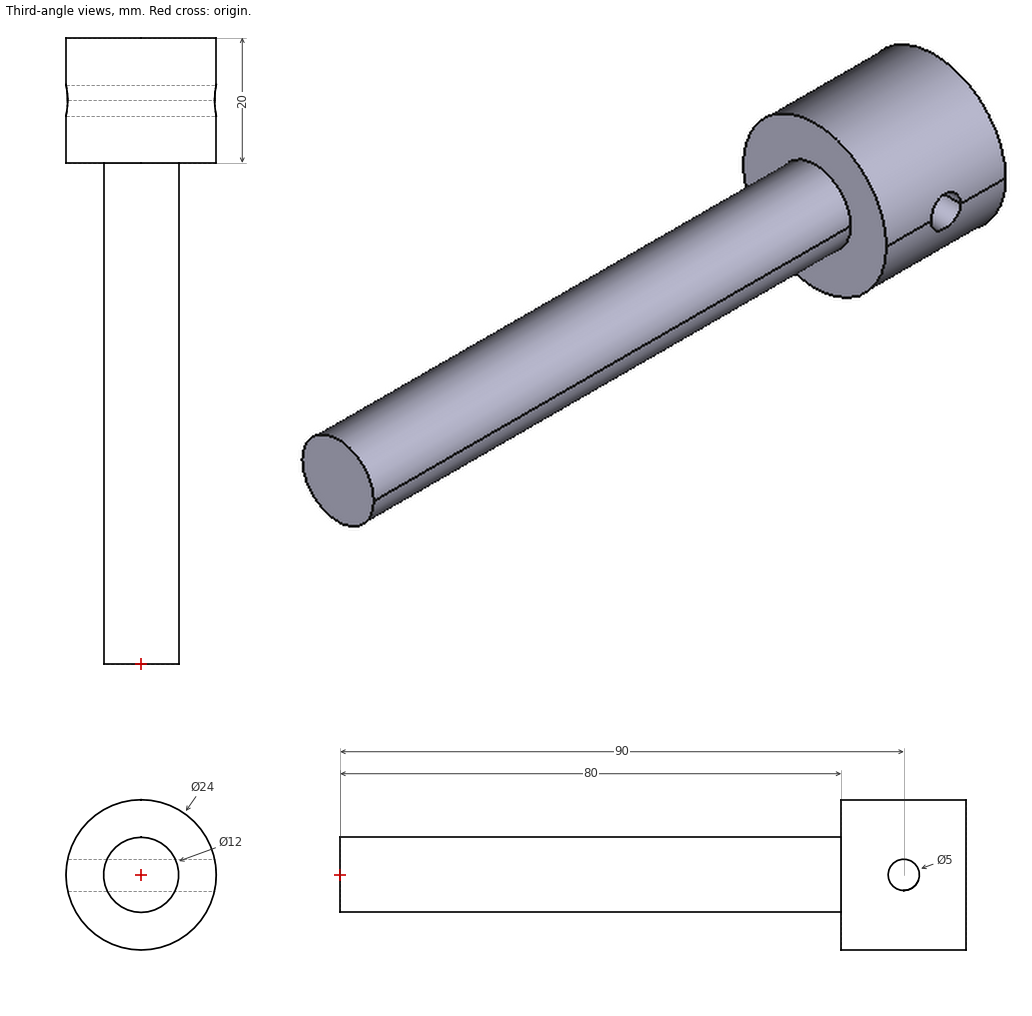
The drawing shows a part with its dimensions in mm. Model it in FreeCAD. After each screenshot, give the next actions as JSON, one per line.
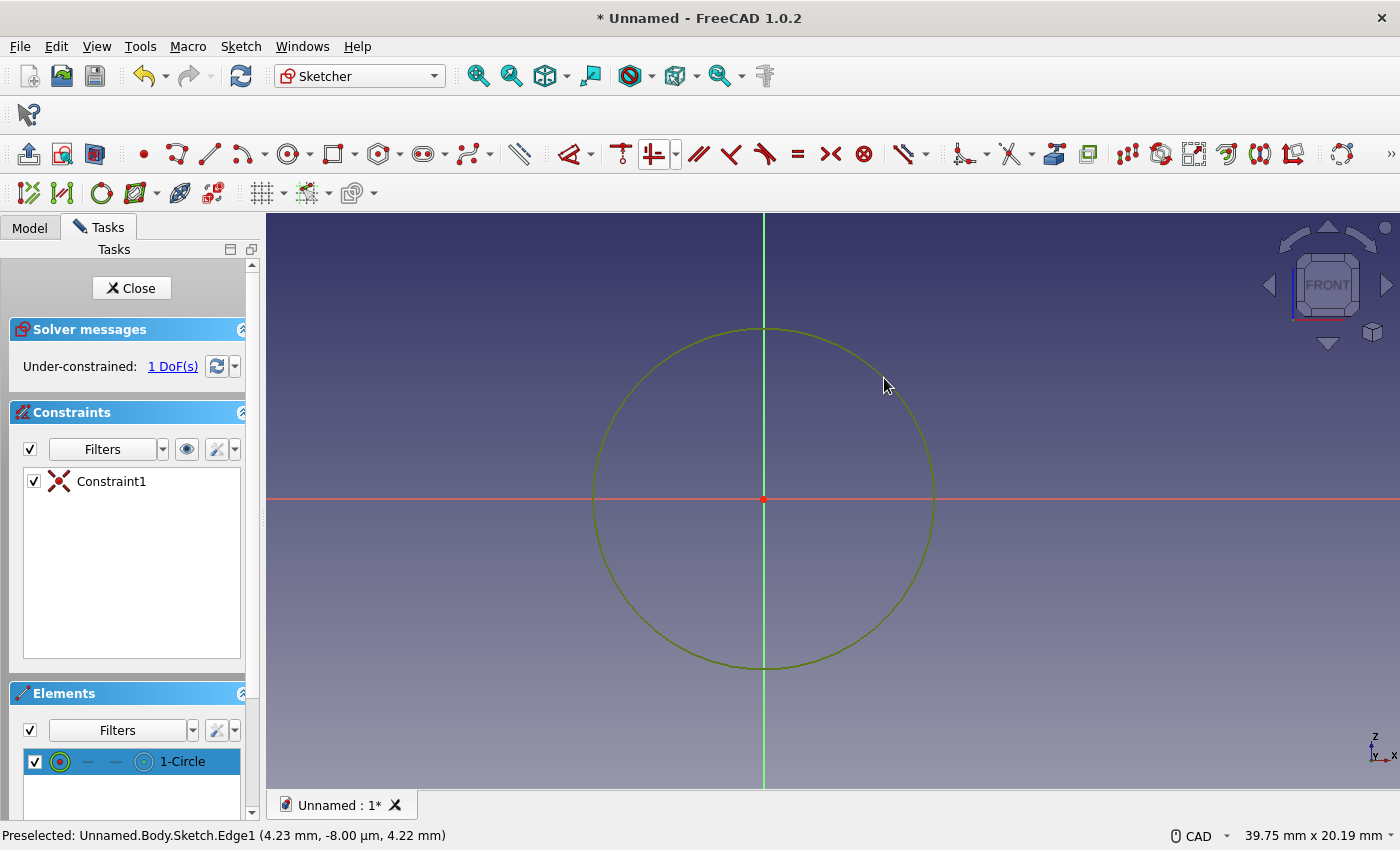
{"action": "key", "text": "k o"}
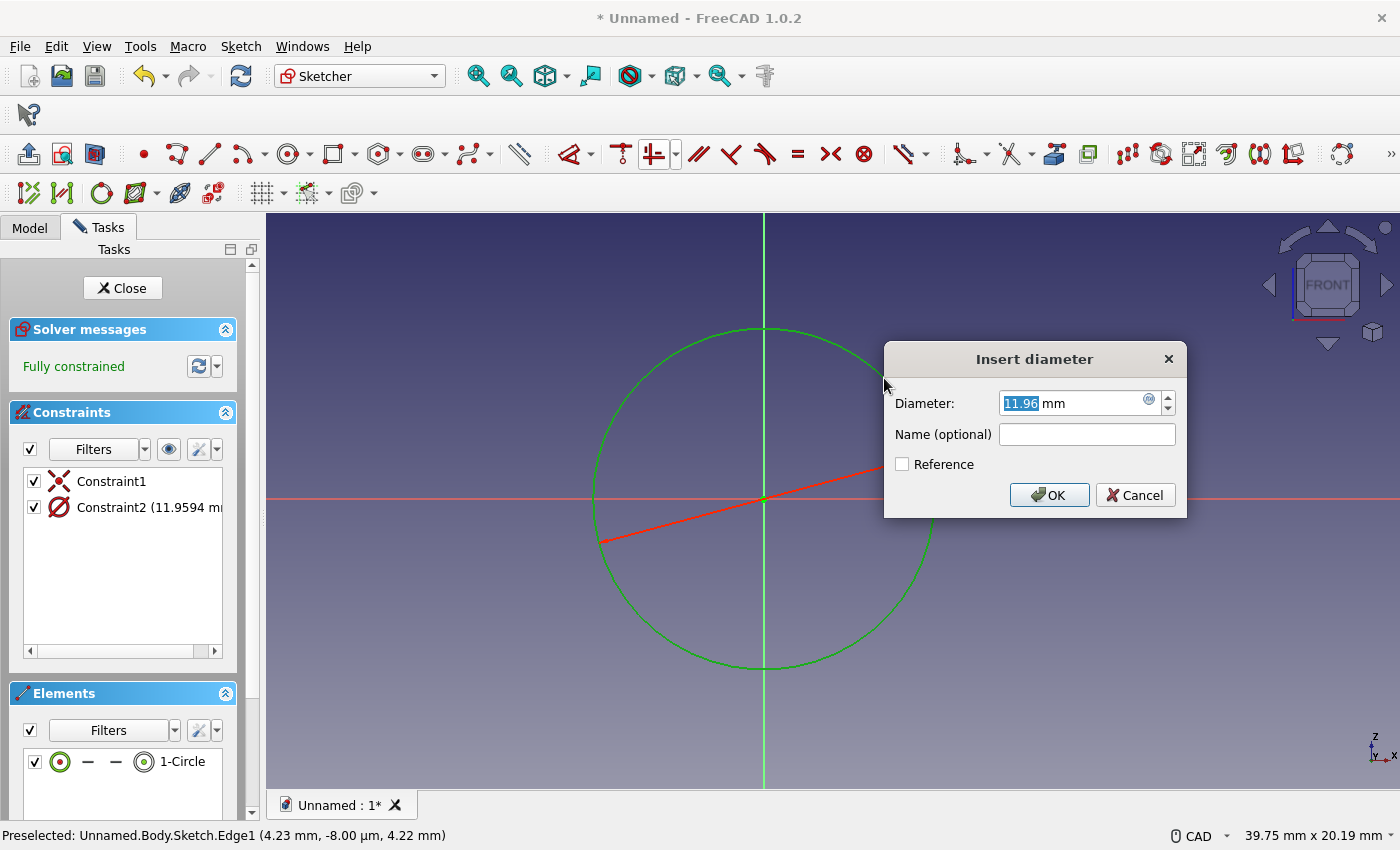
{"action": "type", "text": "12"}
{"action": "key", "text": "Return"}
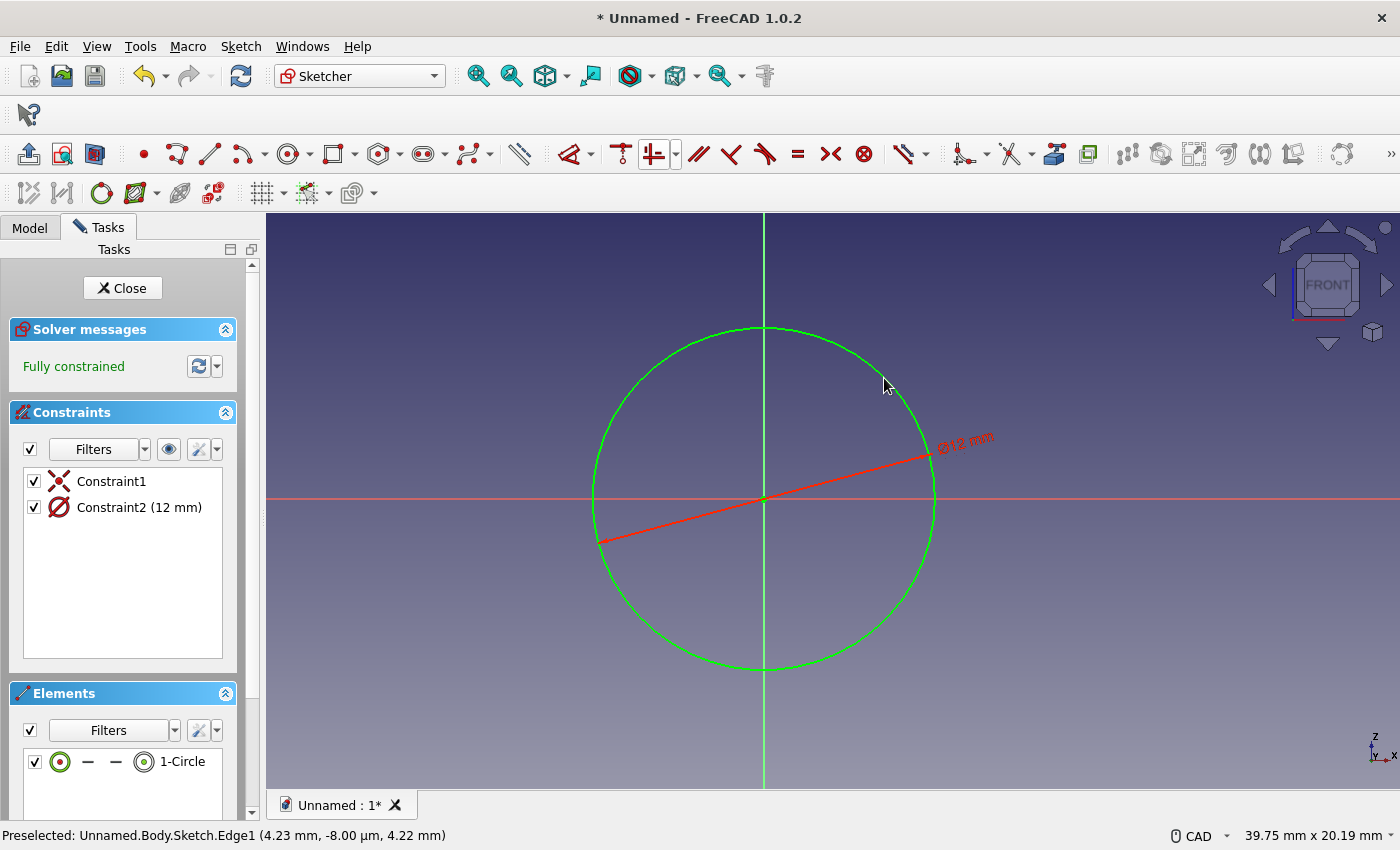
{"action": "left_click", "coordinate": [123, 288]}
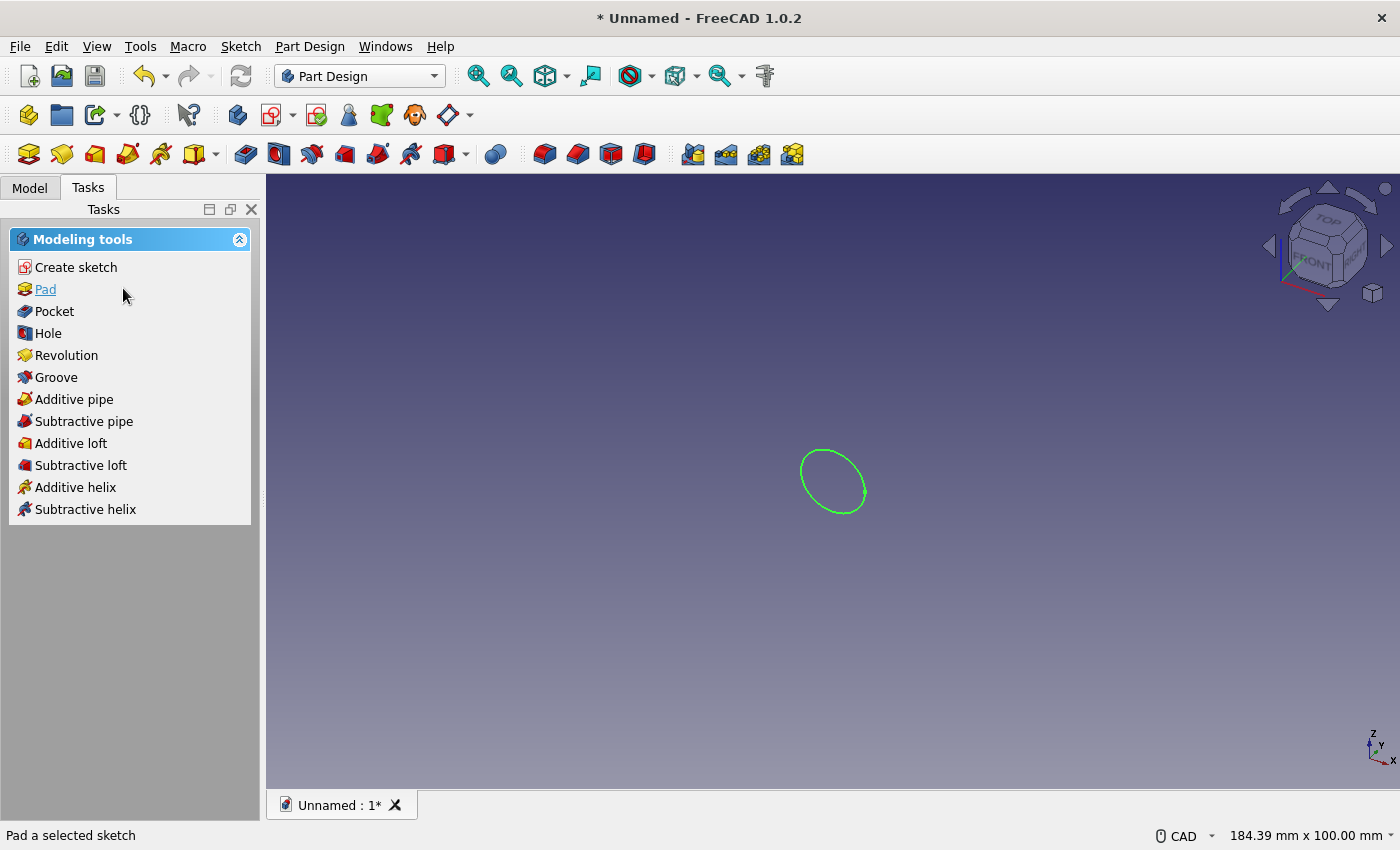
{"action": "left_click", "coordinate": [29, 154]}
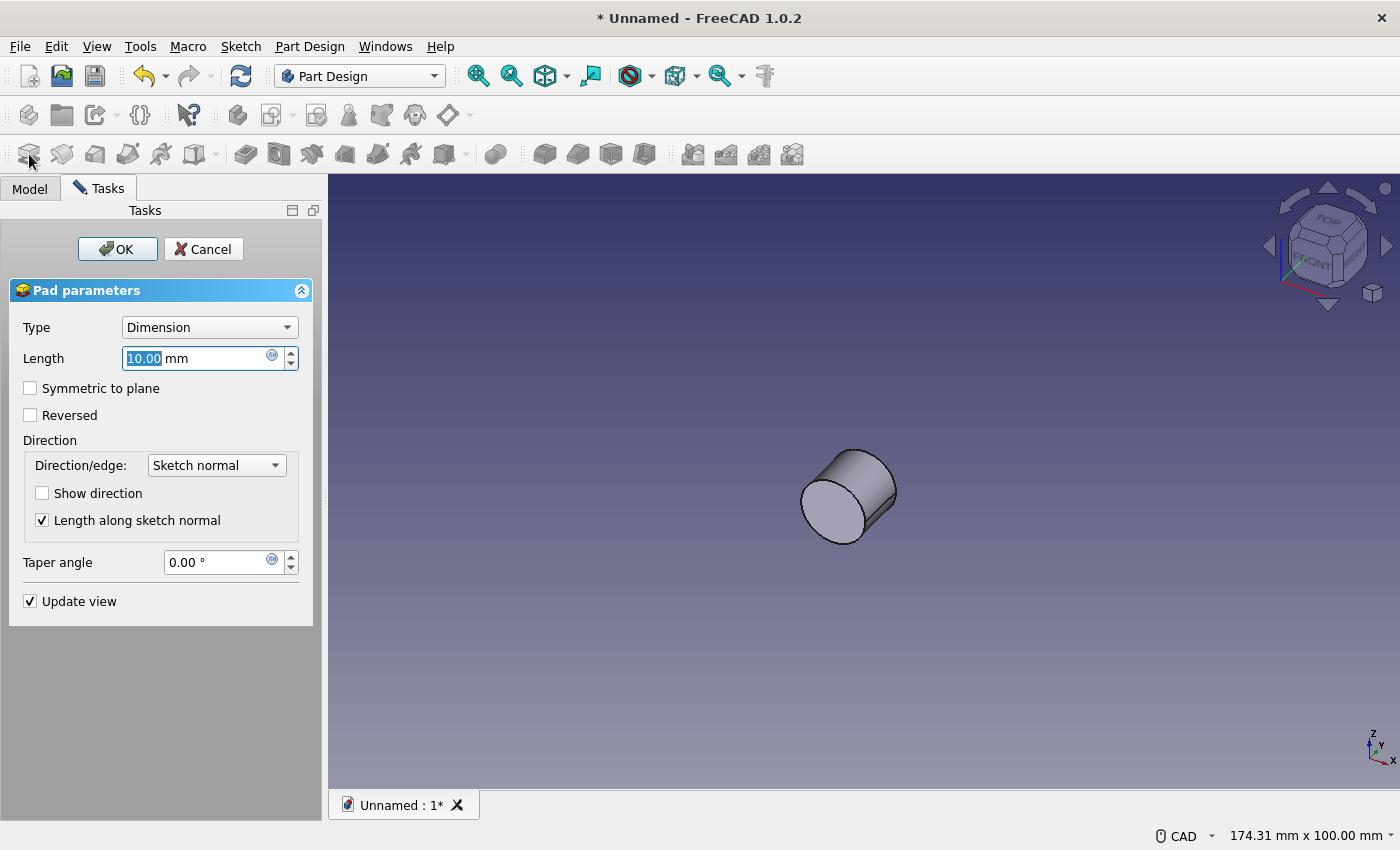
{"action": "type", "text": "80"}
{"action": "key", "text": "Tab"}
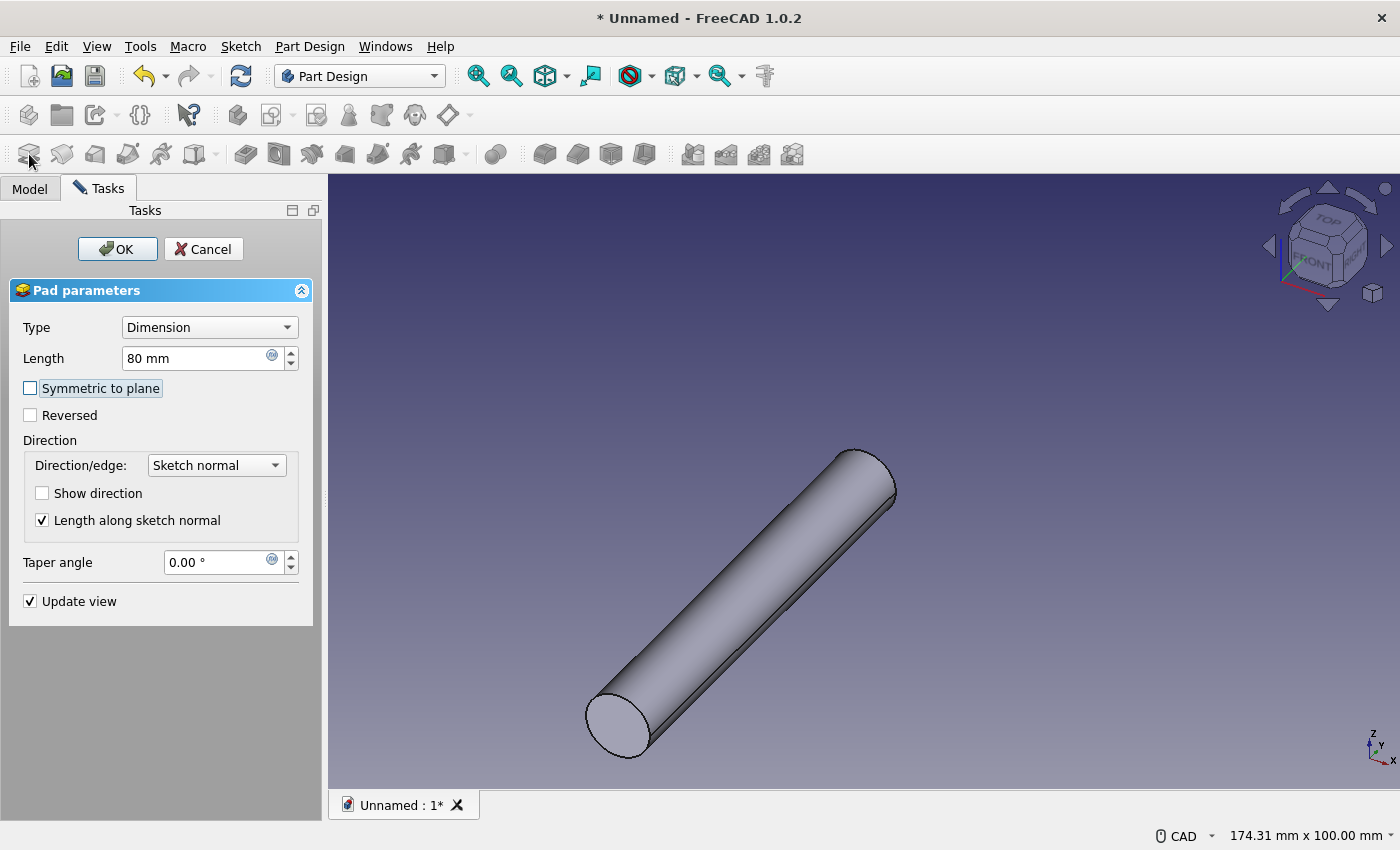
{"action": "left_click", "coordinate": [31, 415]}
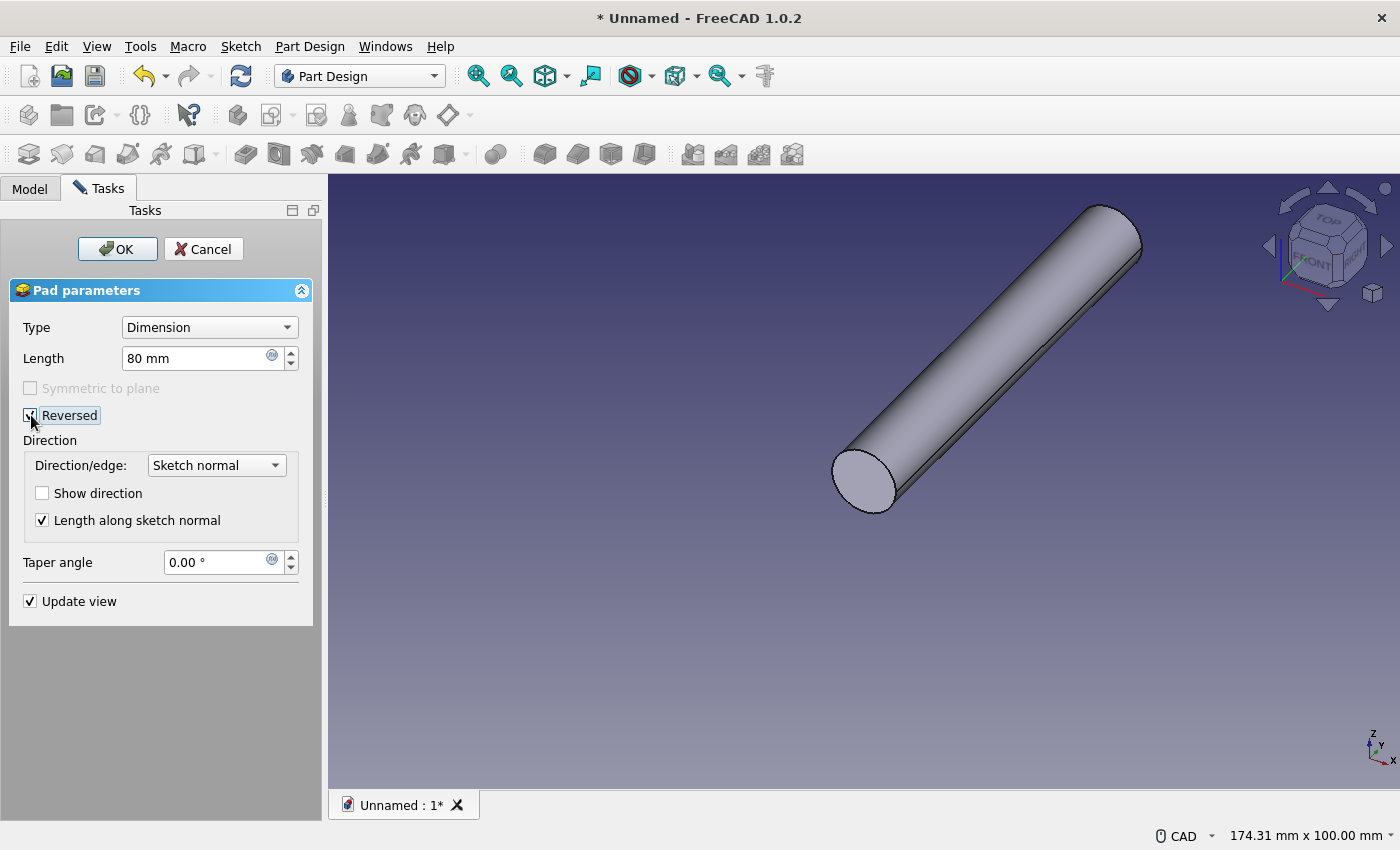
{"action": "left_click", "coordinate": [118, 249]}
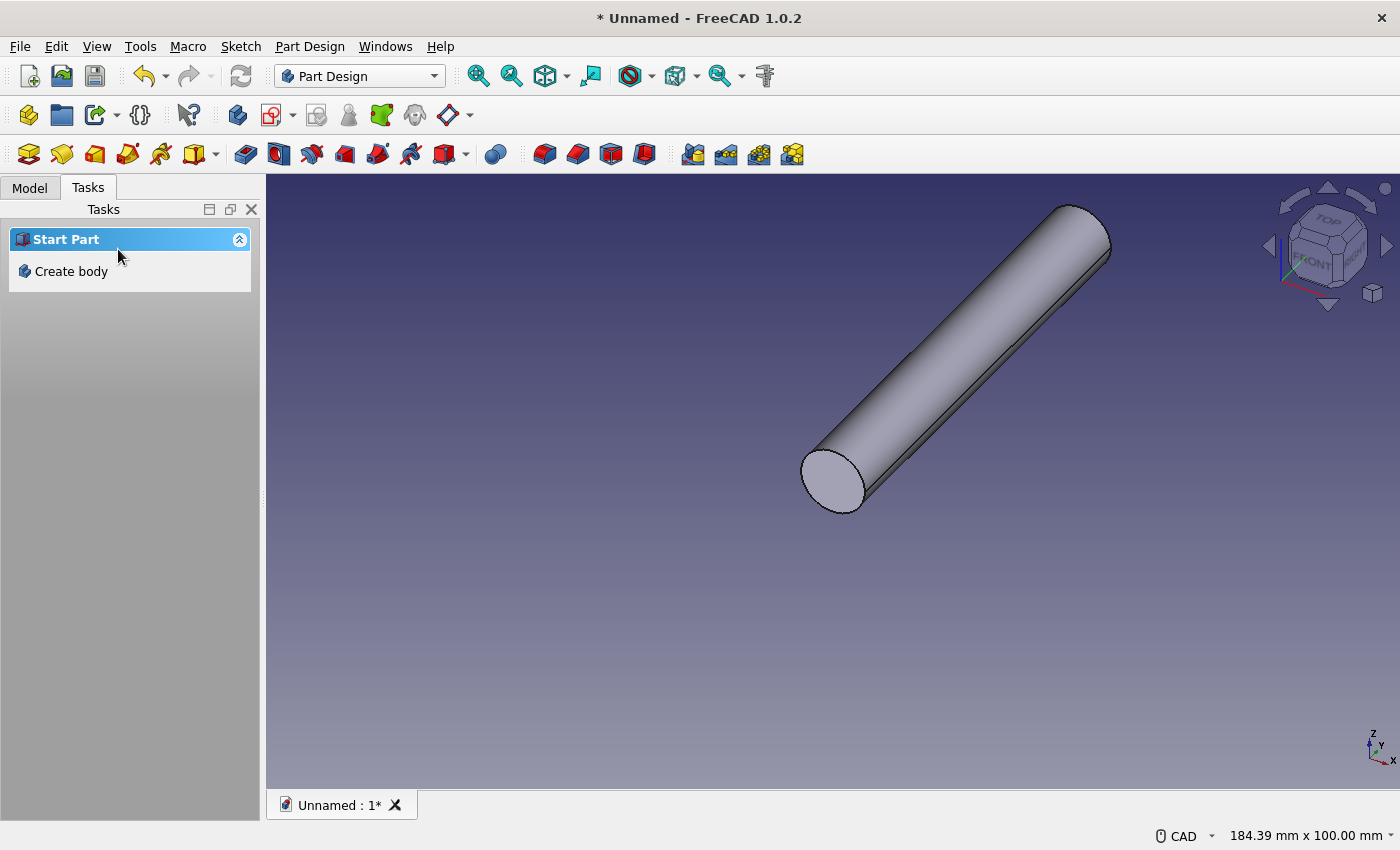
{"action": "key", "text": "4"}